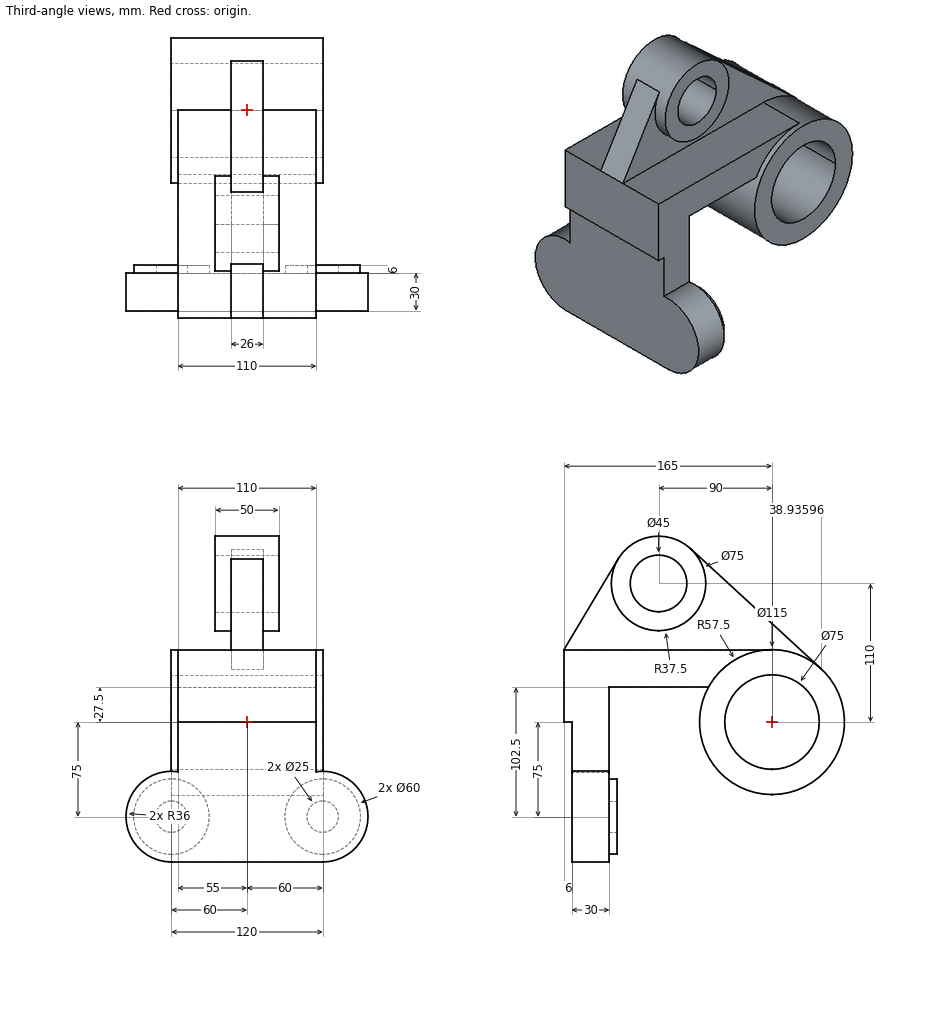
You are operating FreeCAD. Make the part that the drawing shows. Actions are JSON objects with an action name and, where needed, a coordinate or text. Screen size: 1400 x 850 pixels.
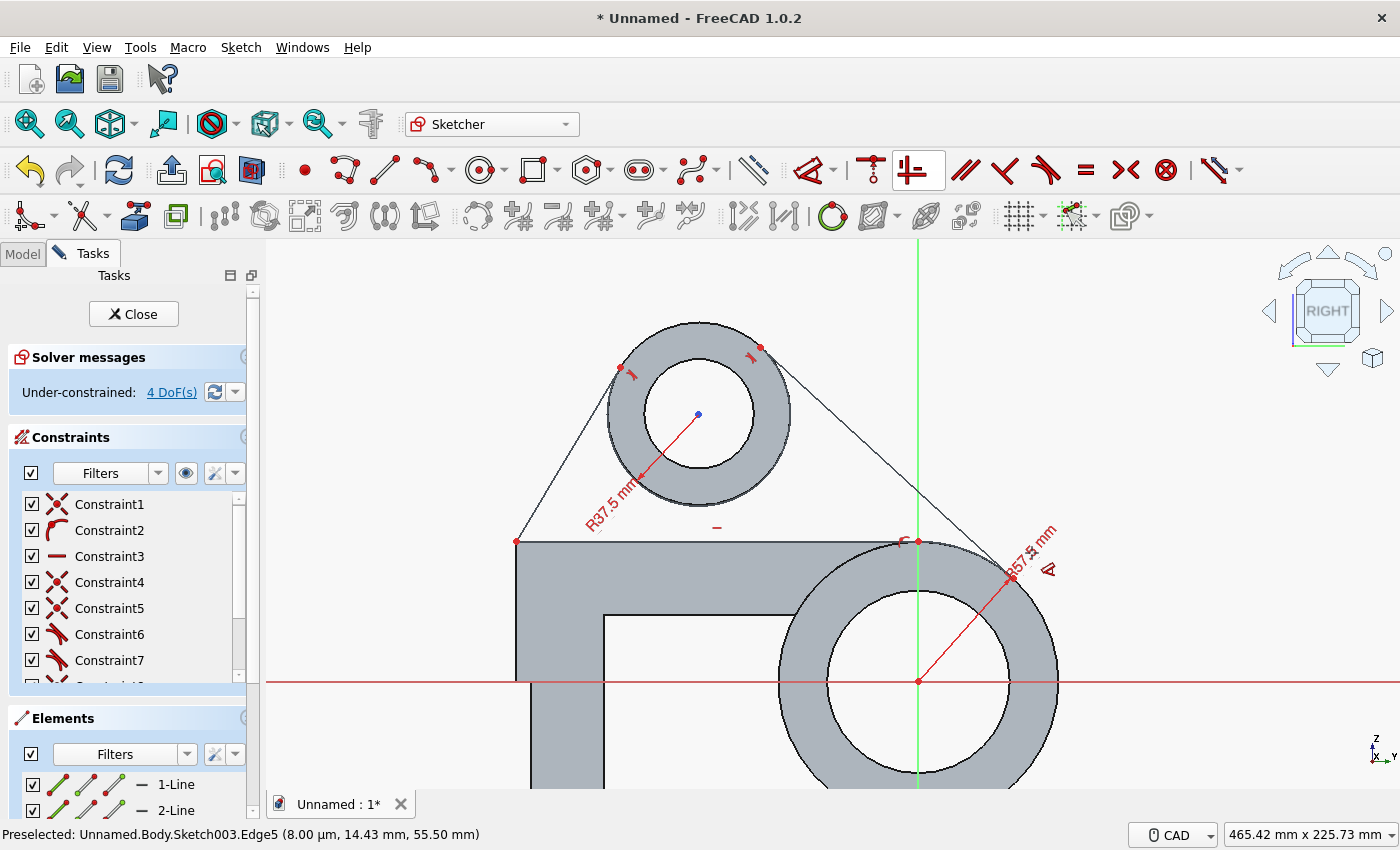
{"action": "left_click", "coordinate": [637, 542]}
{"action": "left_click", "coordinate": [717, 576]}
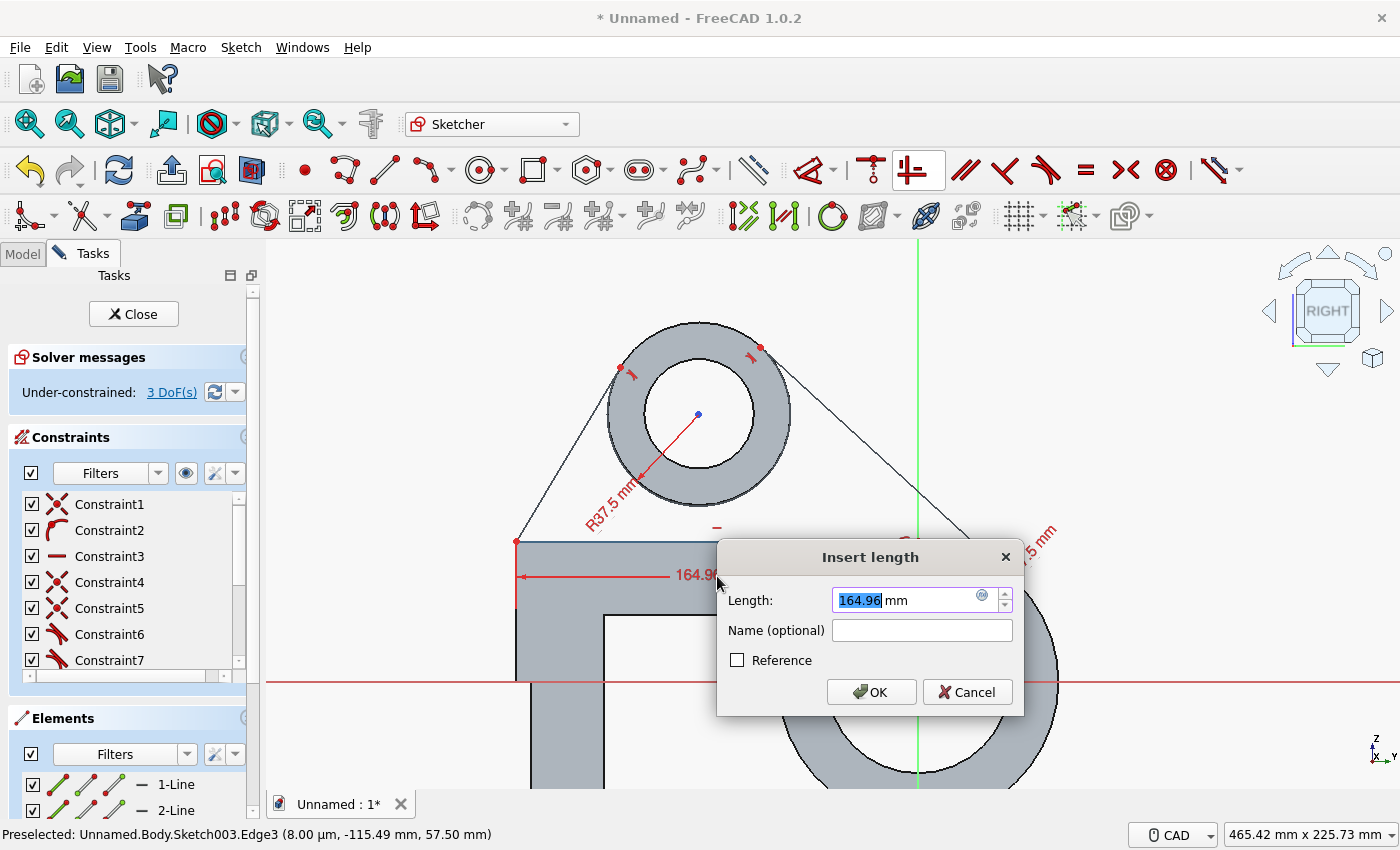
{"action": "type", "text": "165"}
{"action": "key", "text": "Return"}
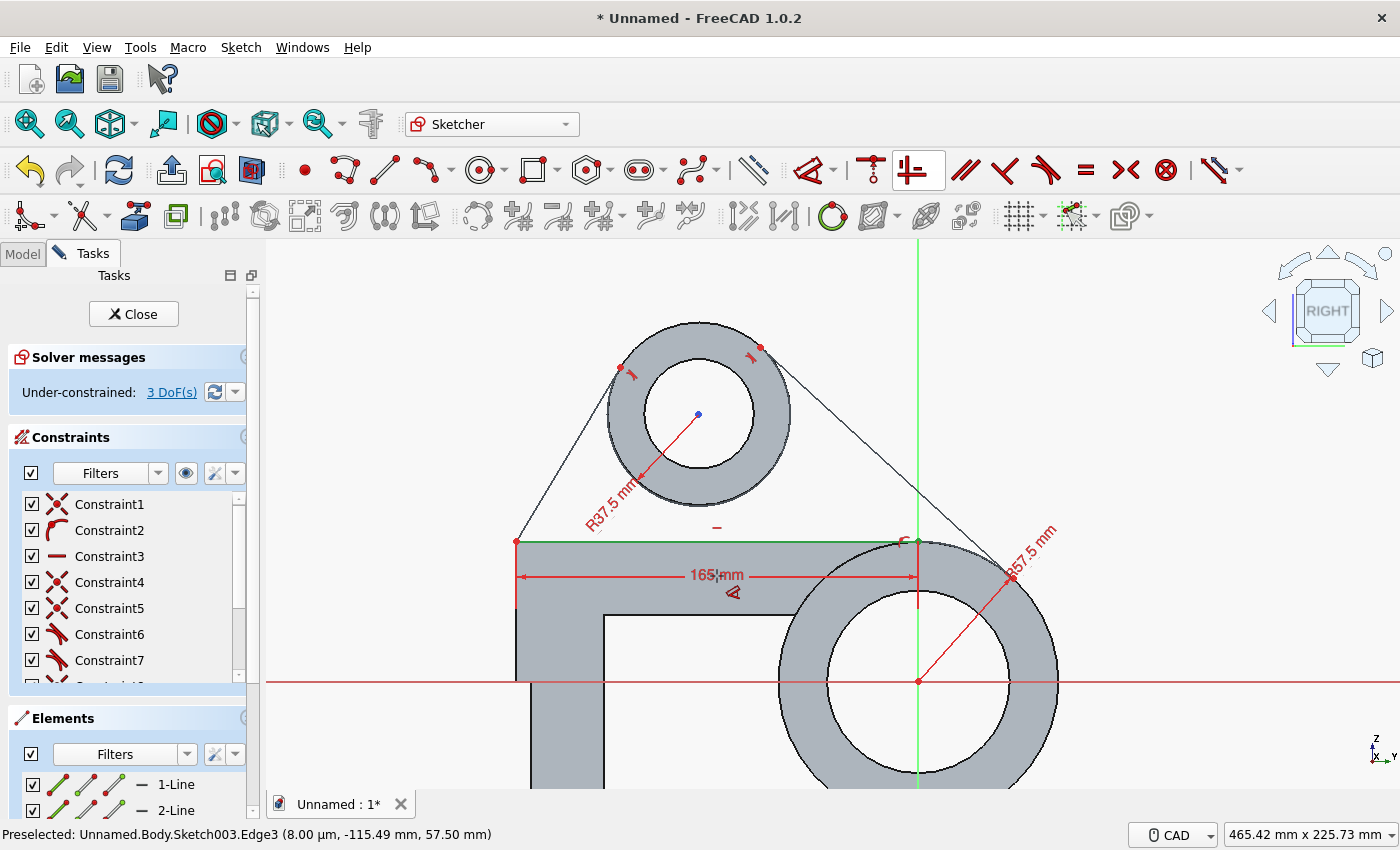
{"action": "left_click", "coordinate": [699, 415]}
{"action": "left_click", "coordinate": [809, 716]}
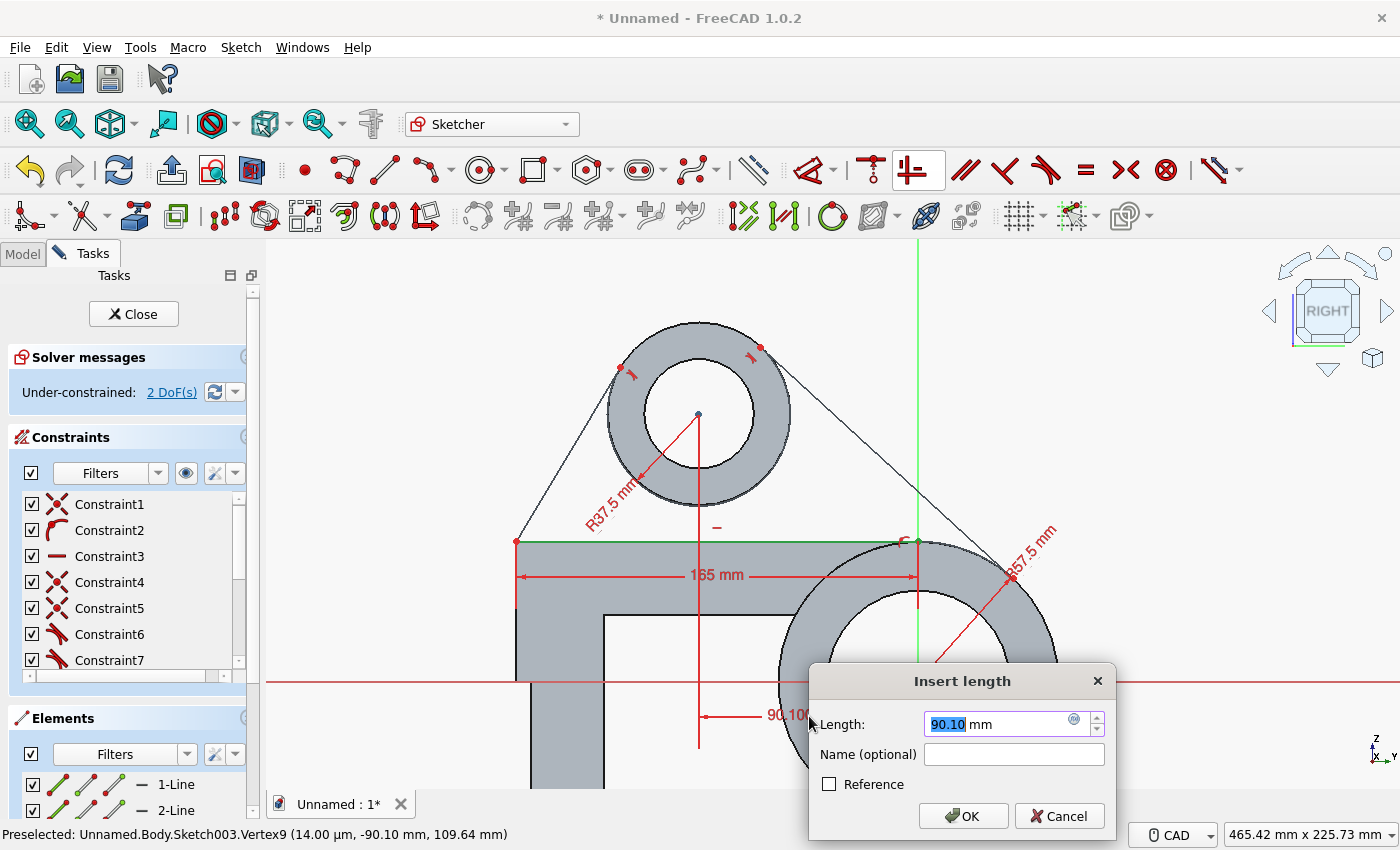
{"action": "type", "text": "90"}
{"action": "key", "text": "Return"}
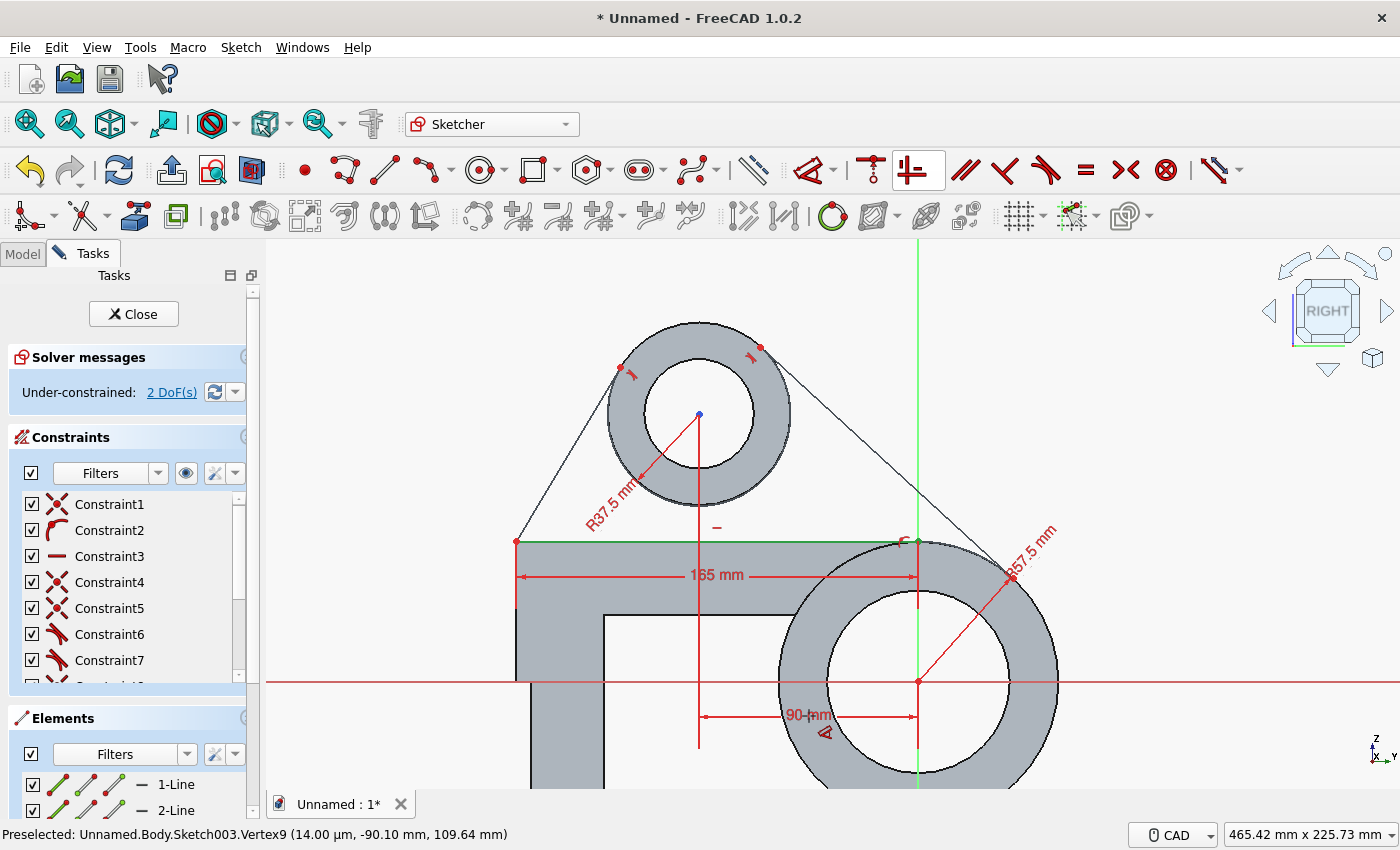
{"action": "left_click", "coordinate": [699, 415]}
{"action": "left_click", "coordinate": [952, 487]}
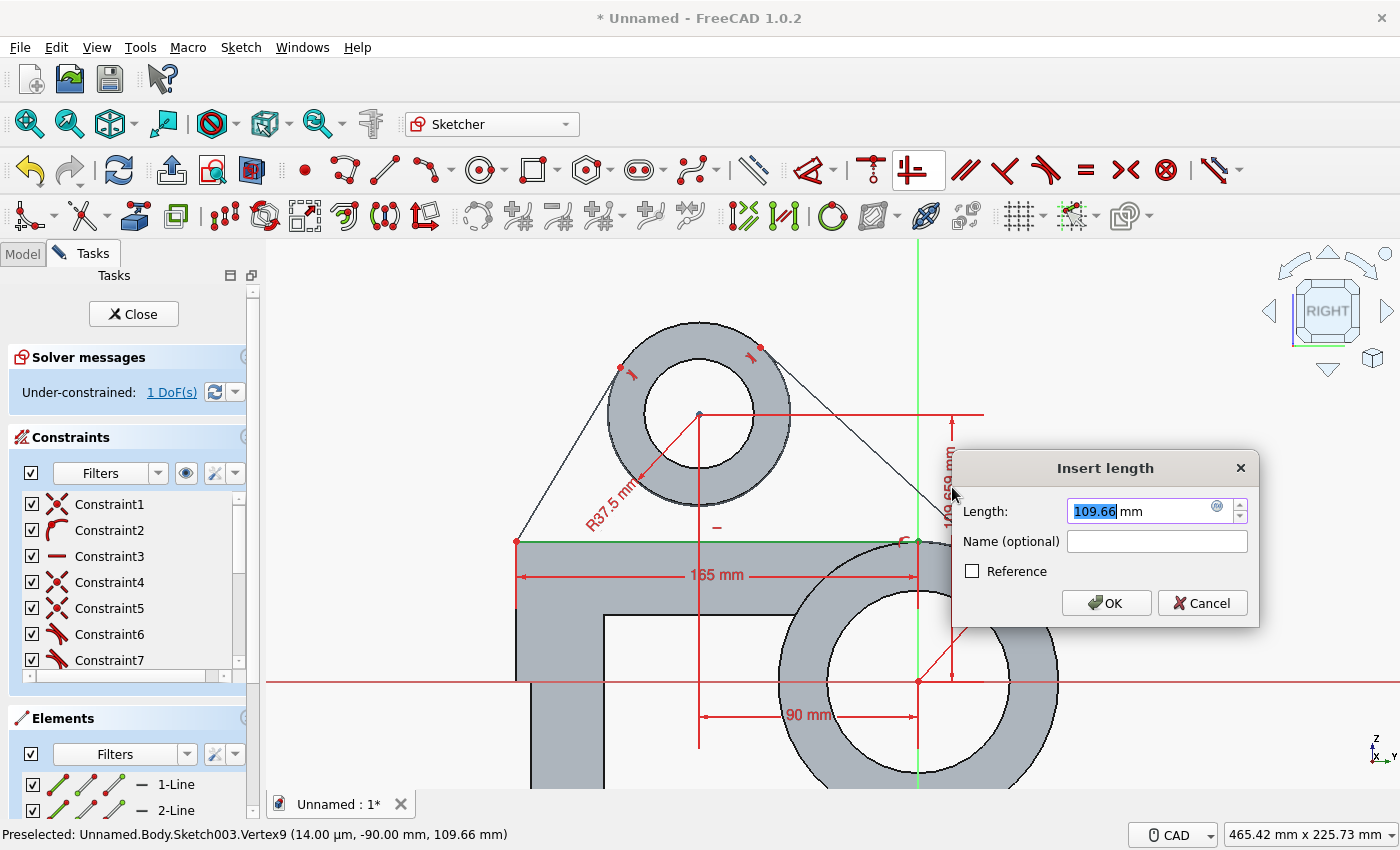
{"action": "type", "text": "110"}
{"action": "key", "text": "Return"}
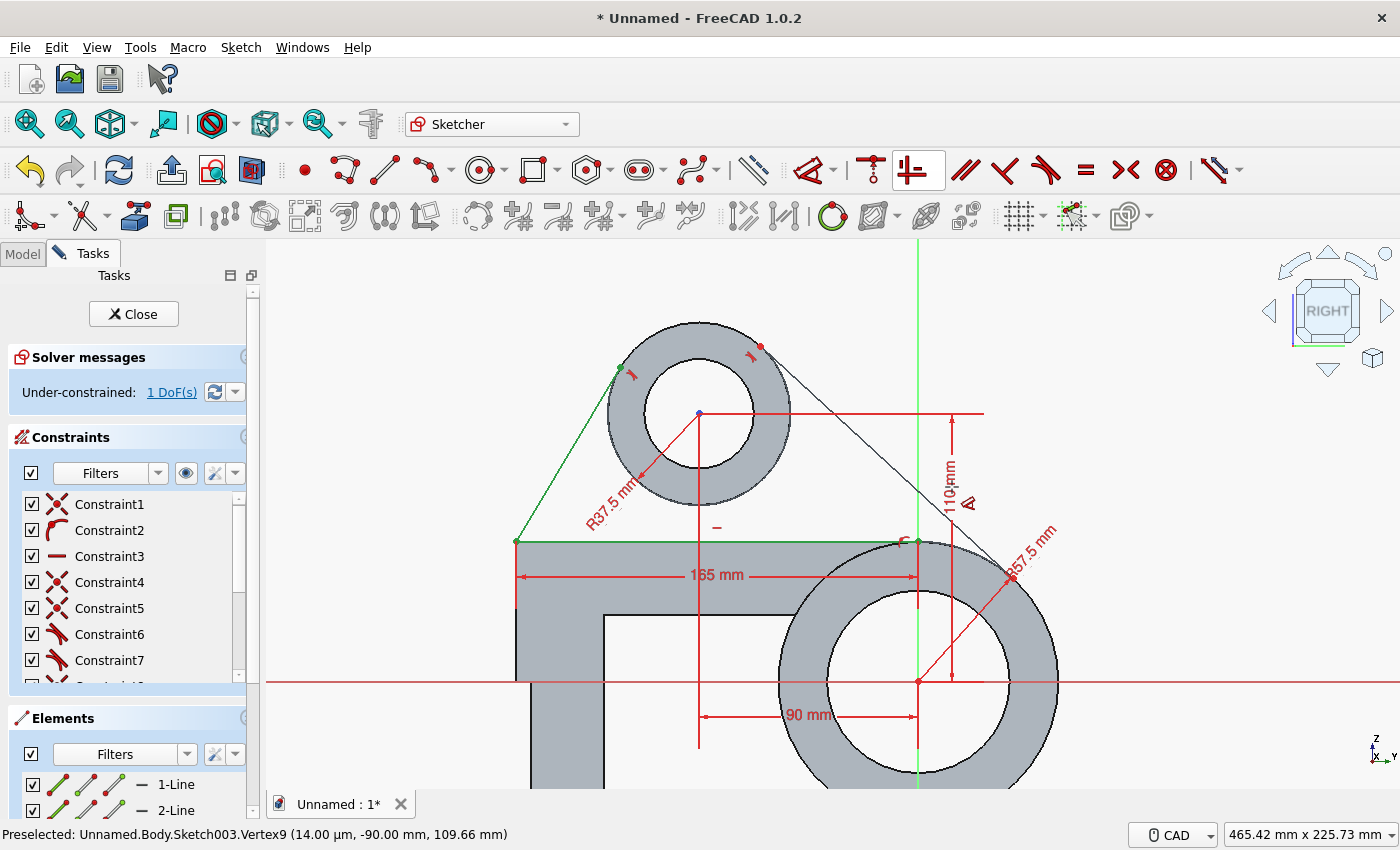
{"action": "left_click", "coordinate": [1013, 579]}
{"action": "left_click", "coordinate": [966, 716]}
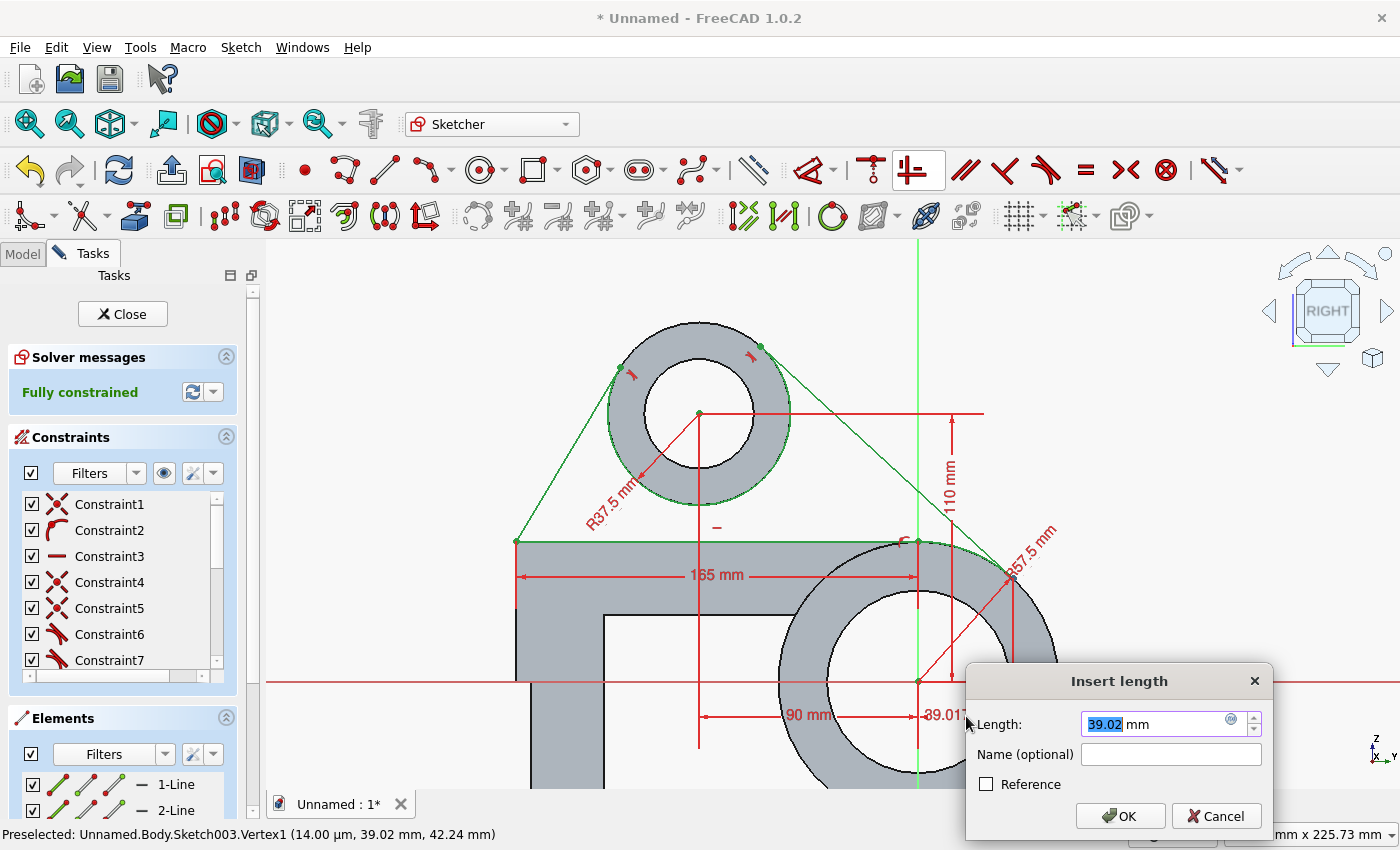
{"action": "type", "text": "38.93596"}
{"action": "key", "text": "Return"}
{"action": "key", "text": "Escape"}